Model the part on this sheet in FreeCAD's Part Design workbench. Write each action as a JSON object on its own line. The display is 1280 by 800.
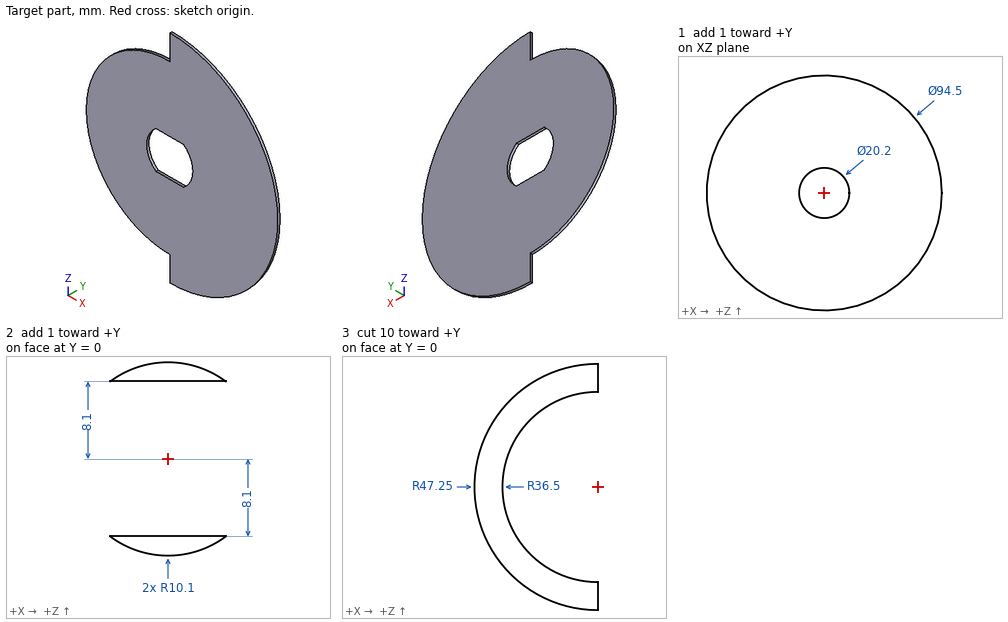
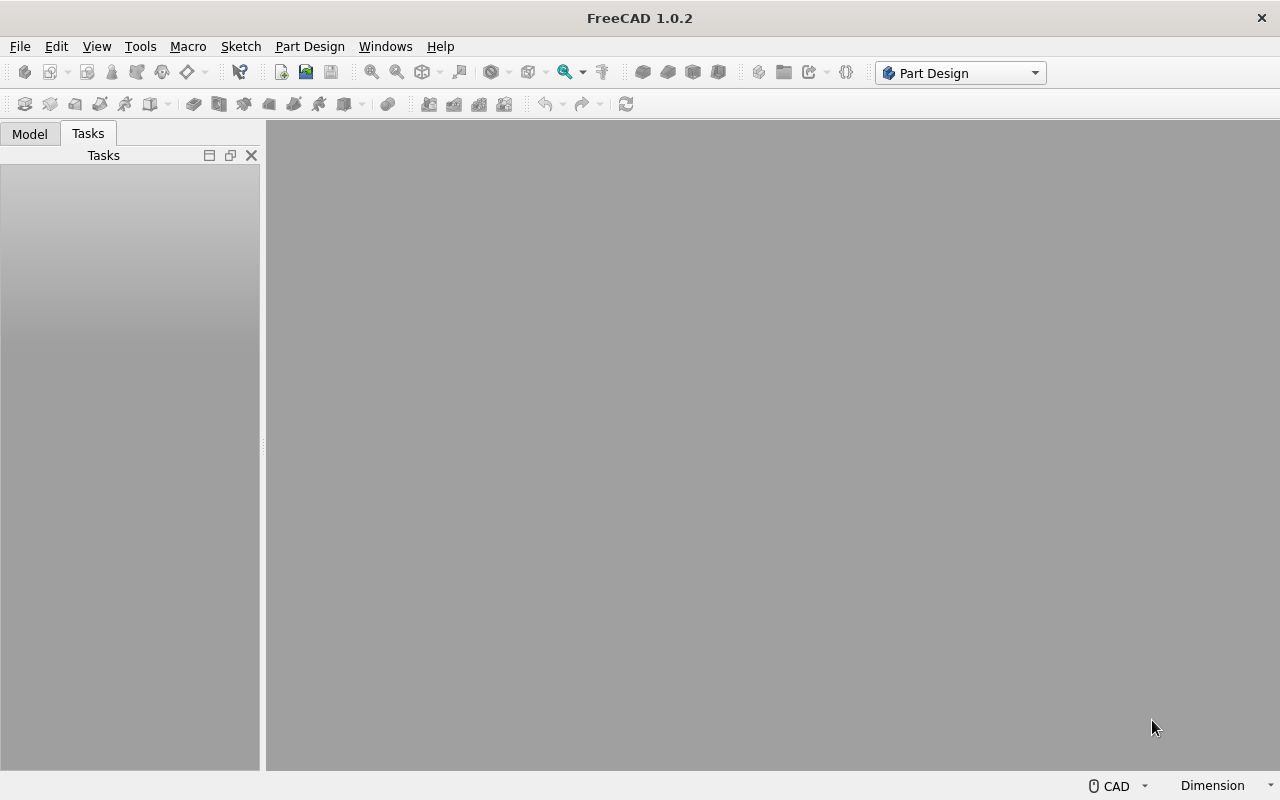
{"action": "left_click", "coordinate": [281, 72]}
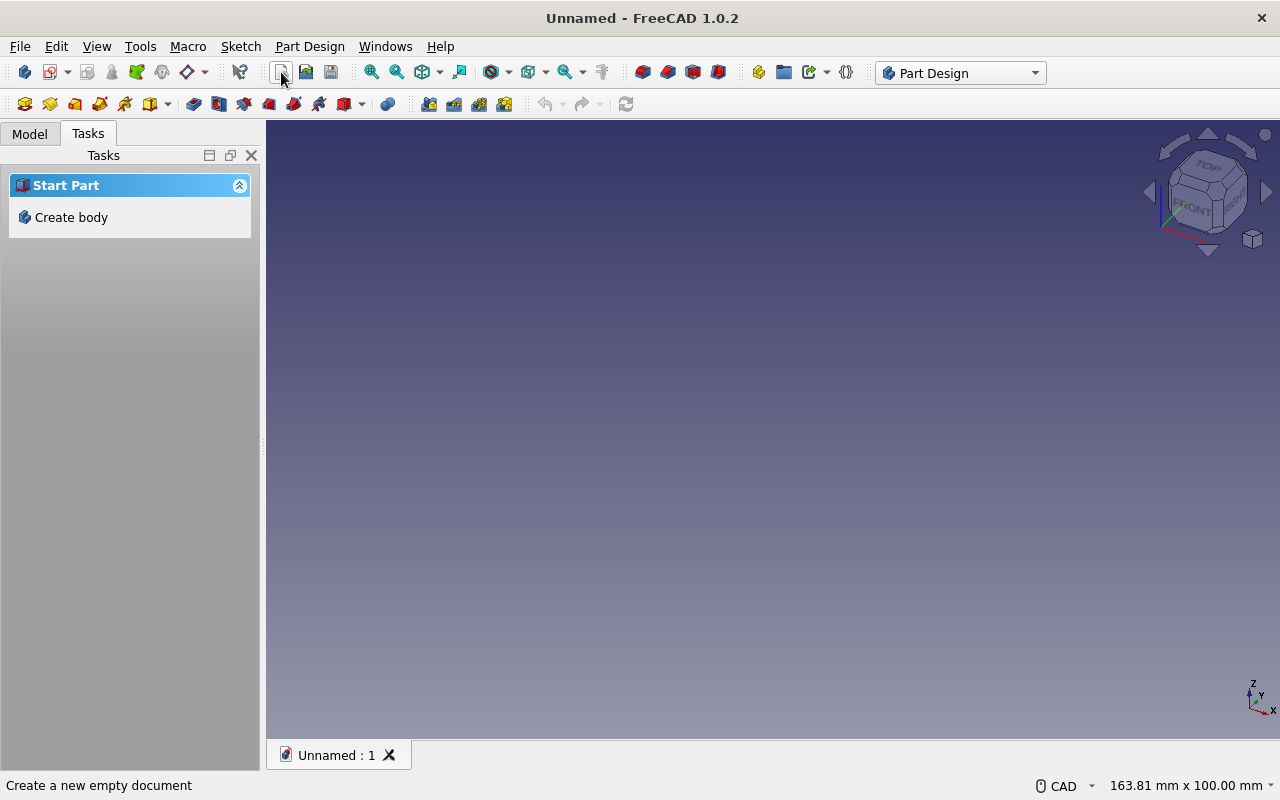
{"action": "left_click", "coordinate": [50, 72]}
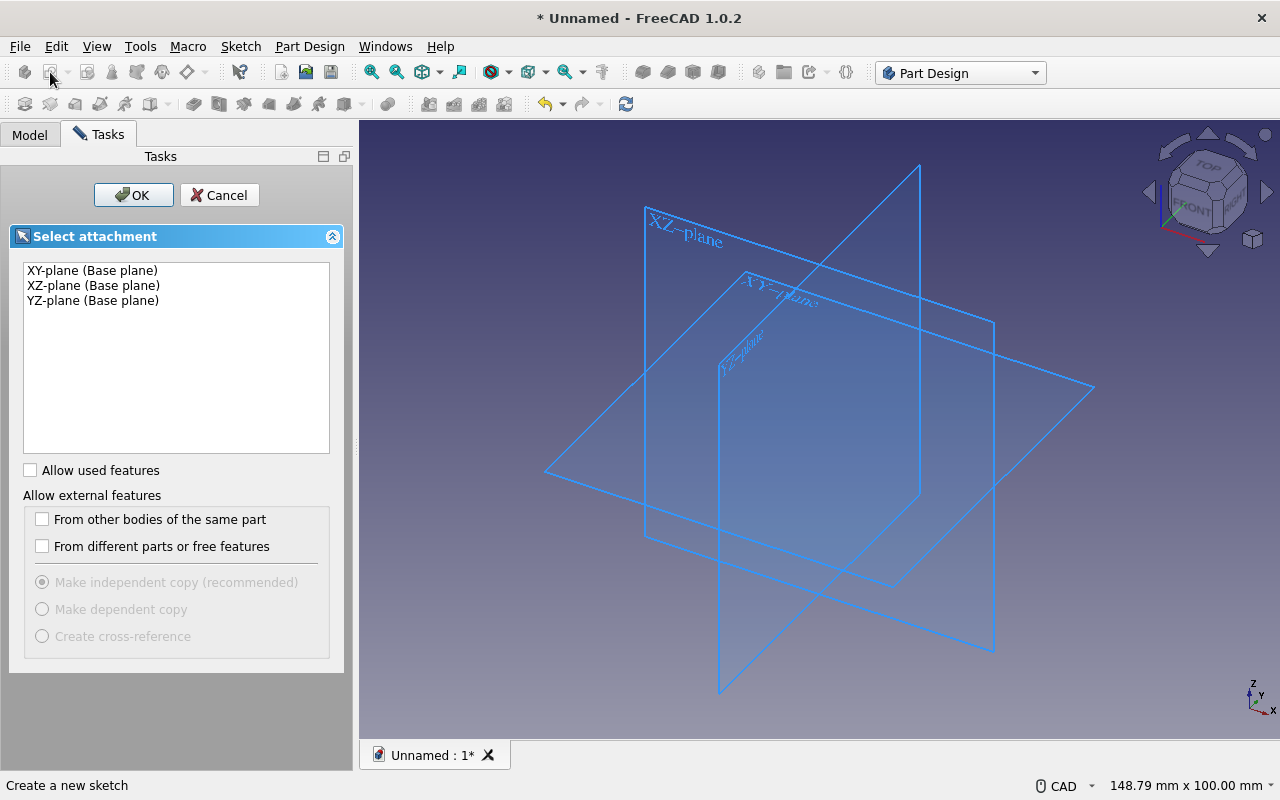
{"action": "left_click", "coordinate": [84, 286]}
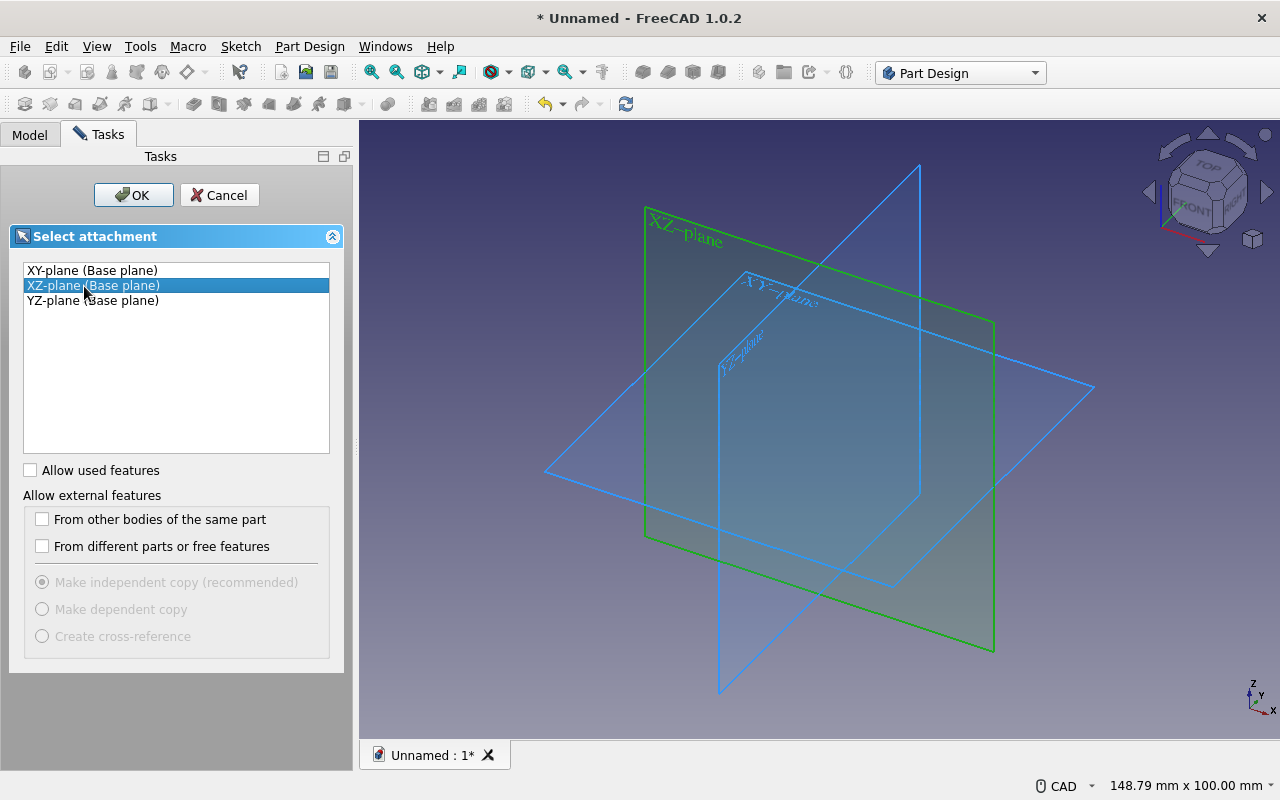
{"action": "left_click", "coordinate": [134, 195]}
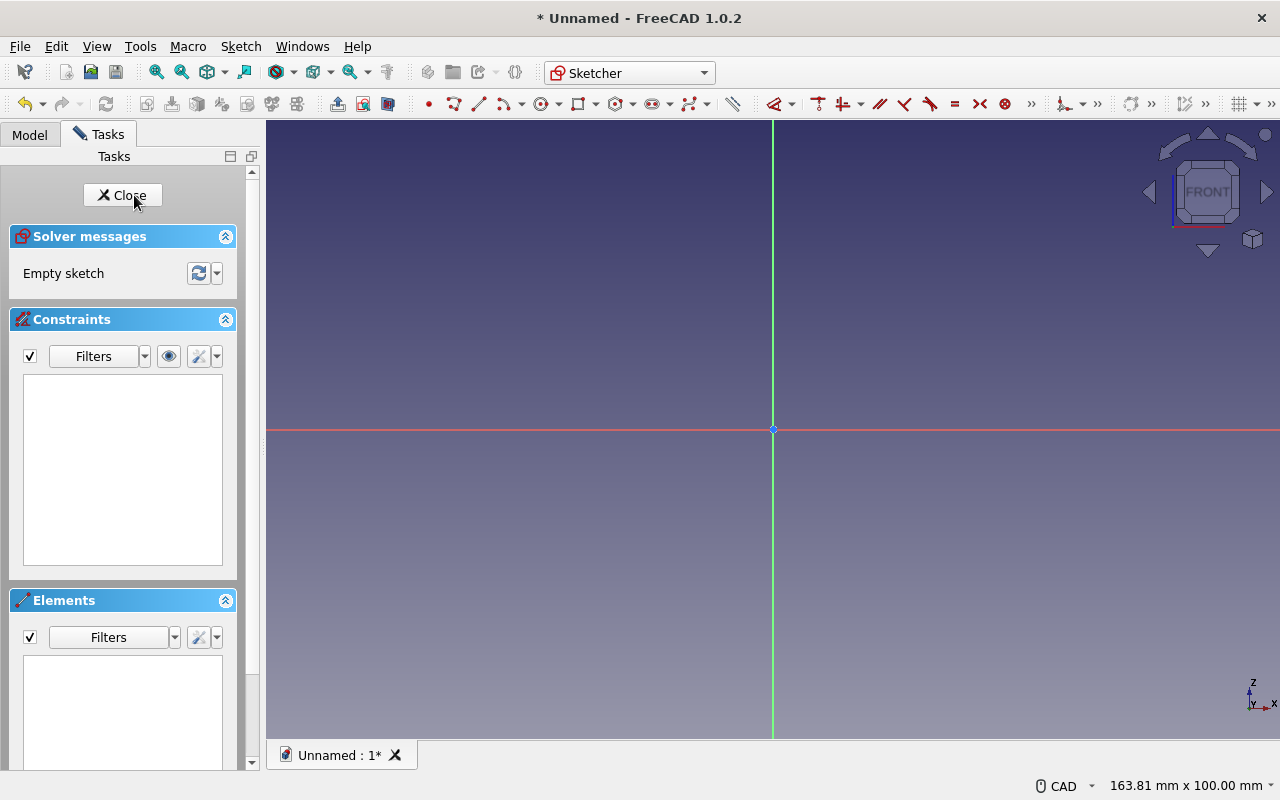
{"action": "scroll", "coordinate": [565, 429], "scroll_direction": "down", "scroll_amount": 2}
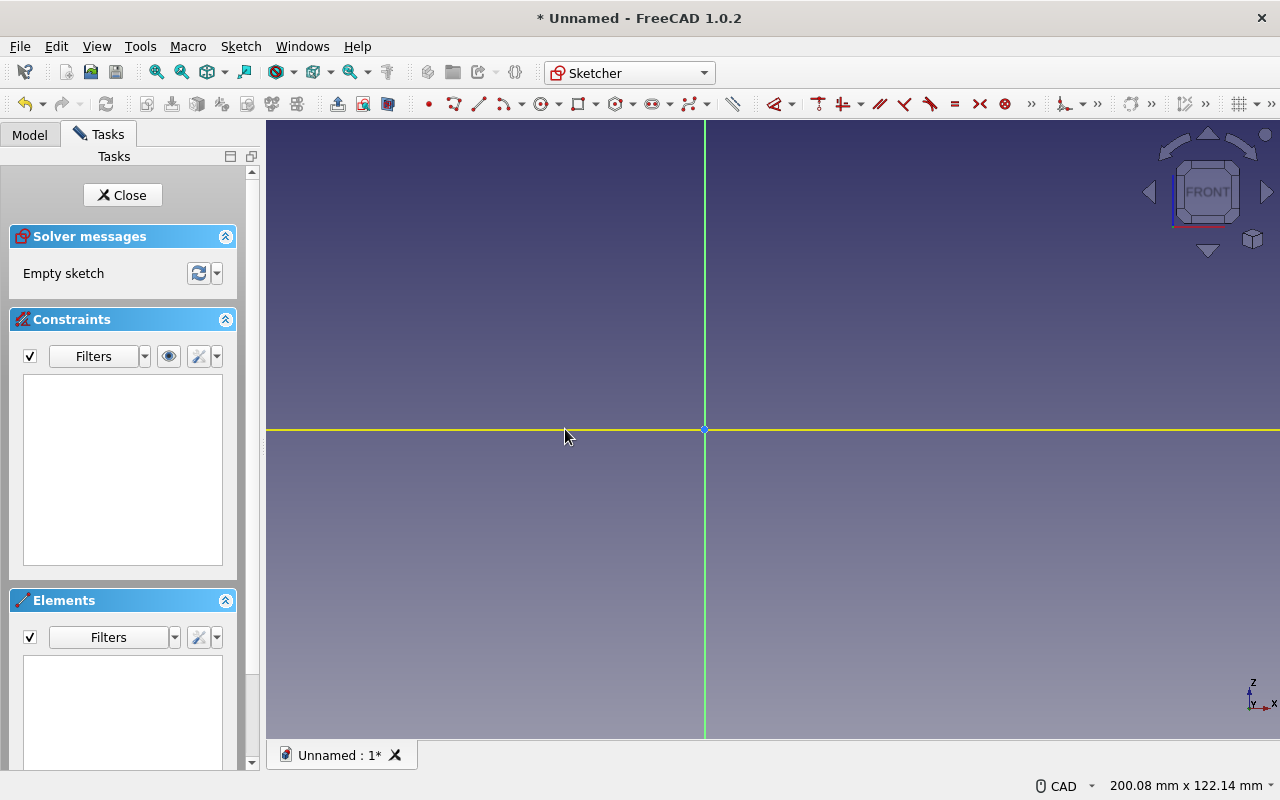
{"action": "left_click", "coordinate": [540, 104]}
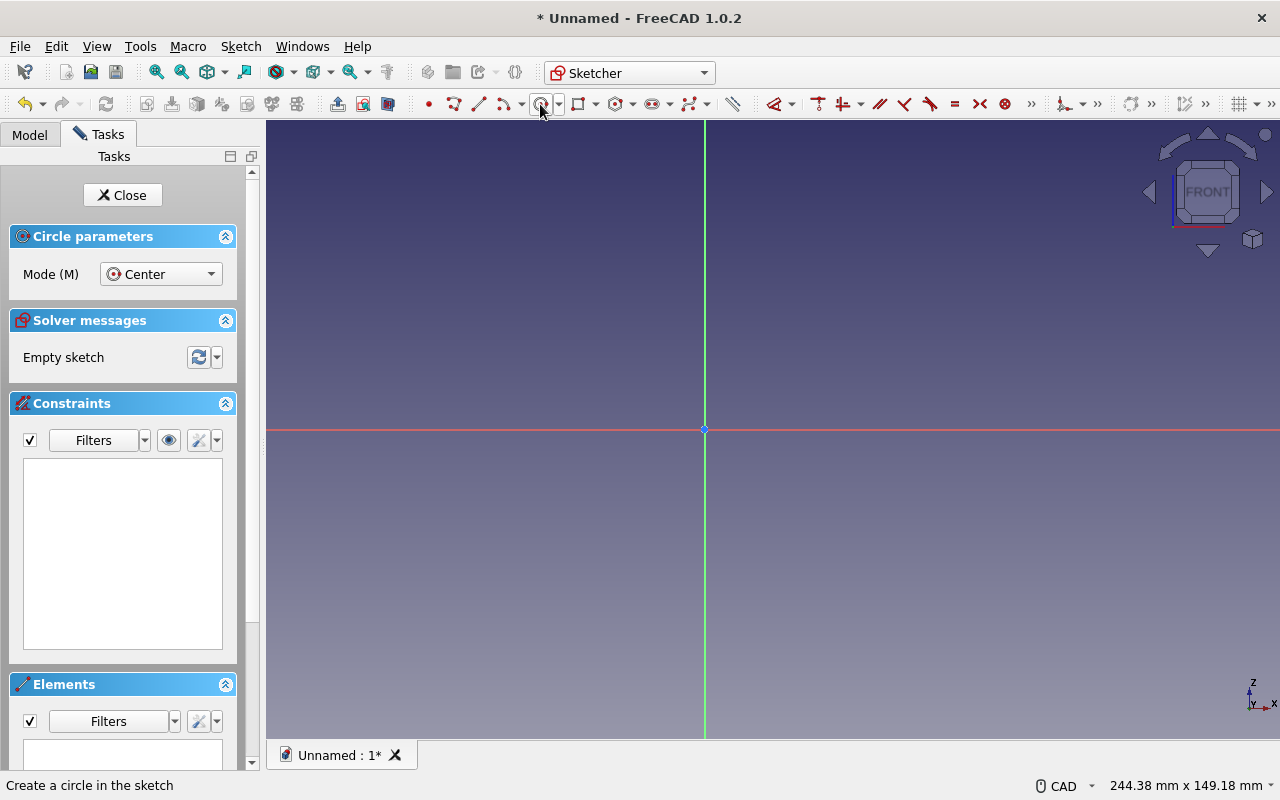
{"action": "left_click", "coordinate": [705, 430]}
{"action": "mouse_move", "coordinate": [843, 291]}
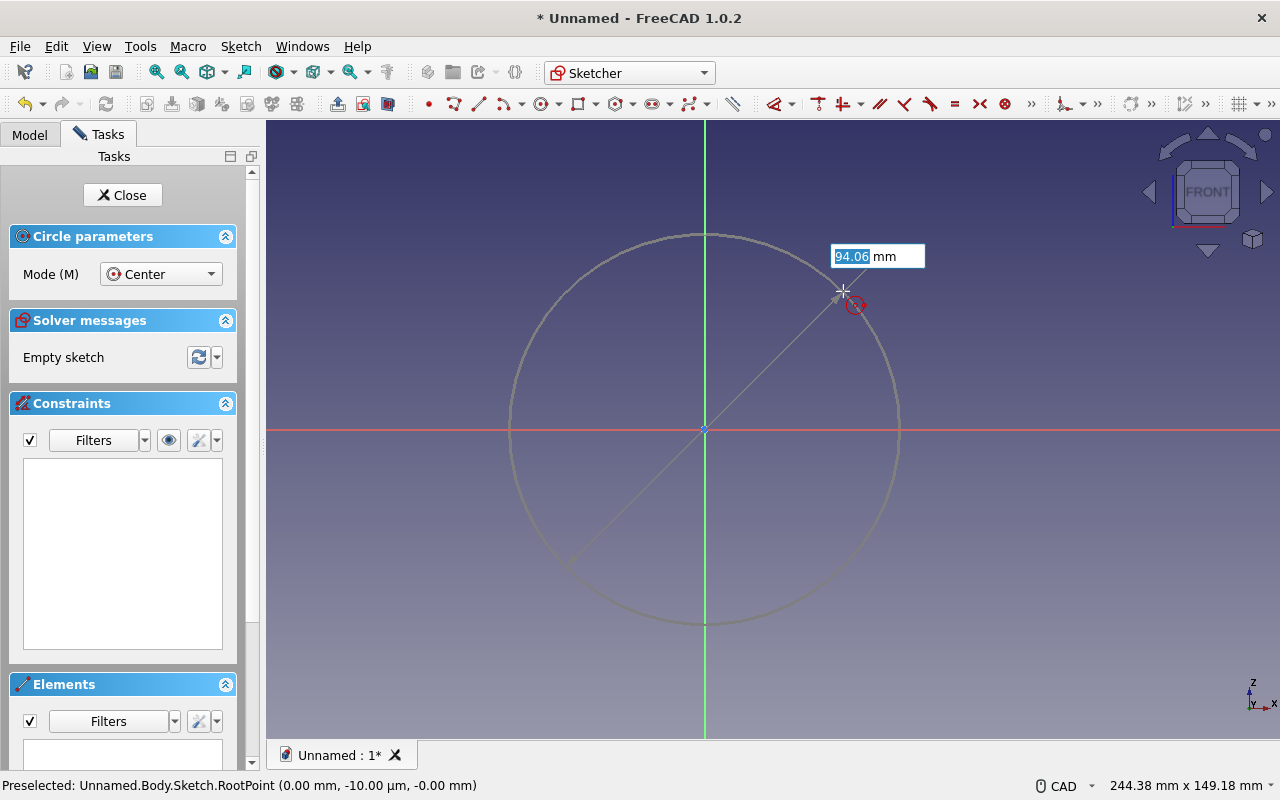
{"action": "type", "text": "94.5"}
{"action": "key", "text": "Return"}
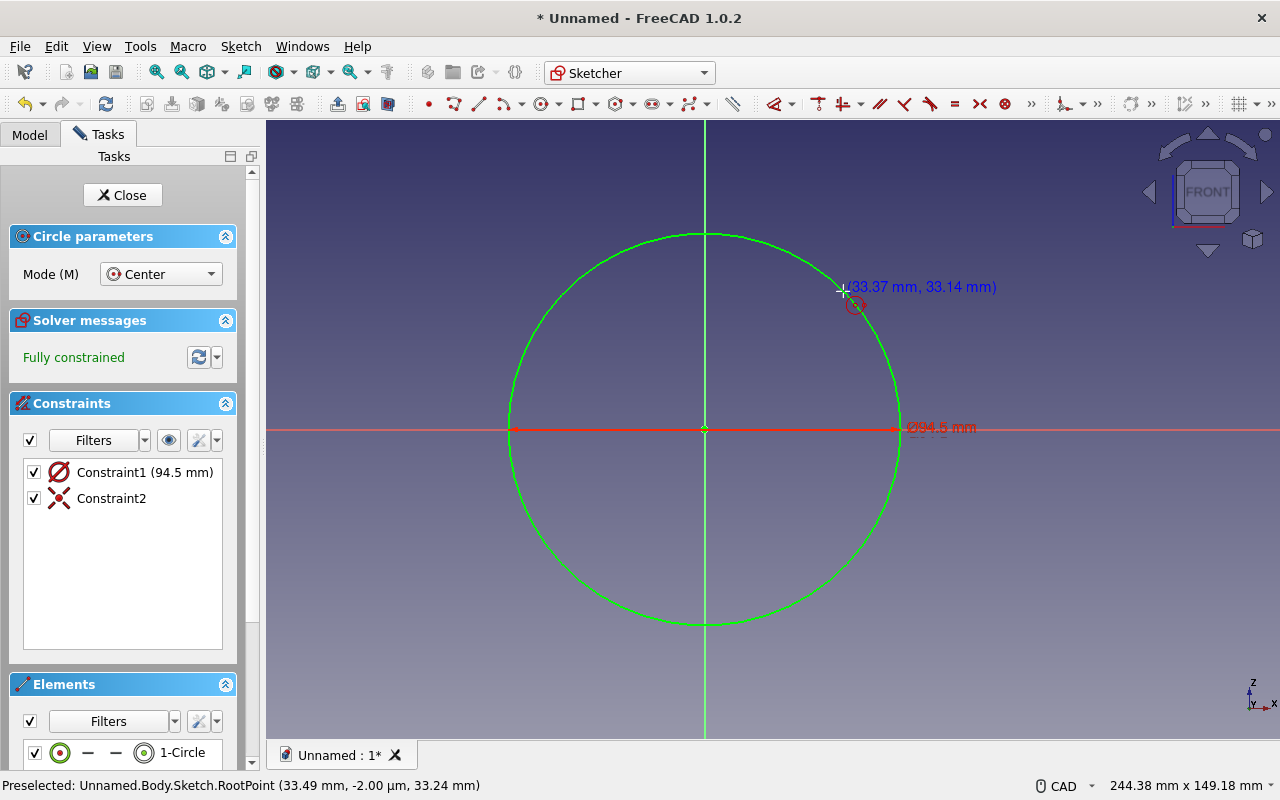
{"action": "left_click", "coordinate": [705, 430]}
{"action": "mouse_move", "coordinate": [734, 400]}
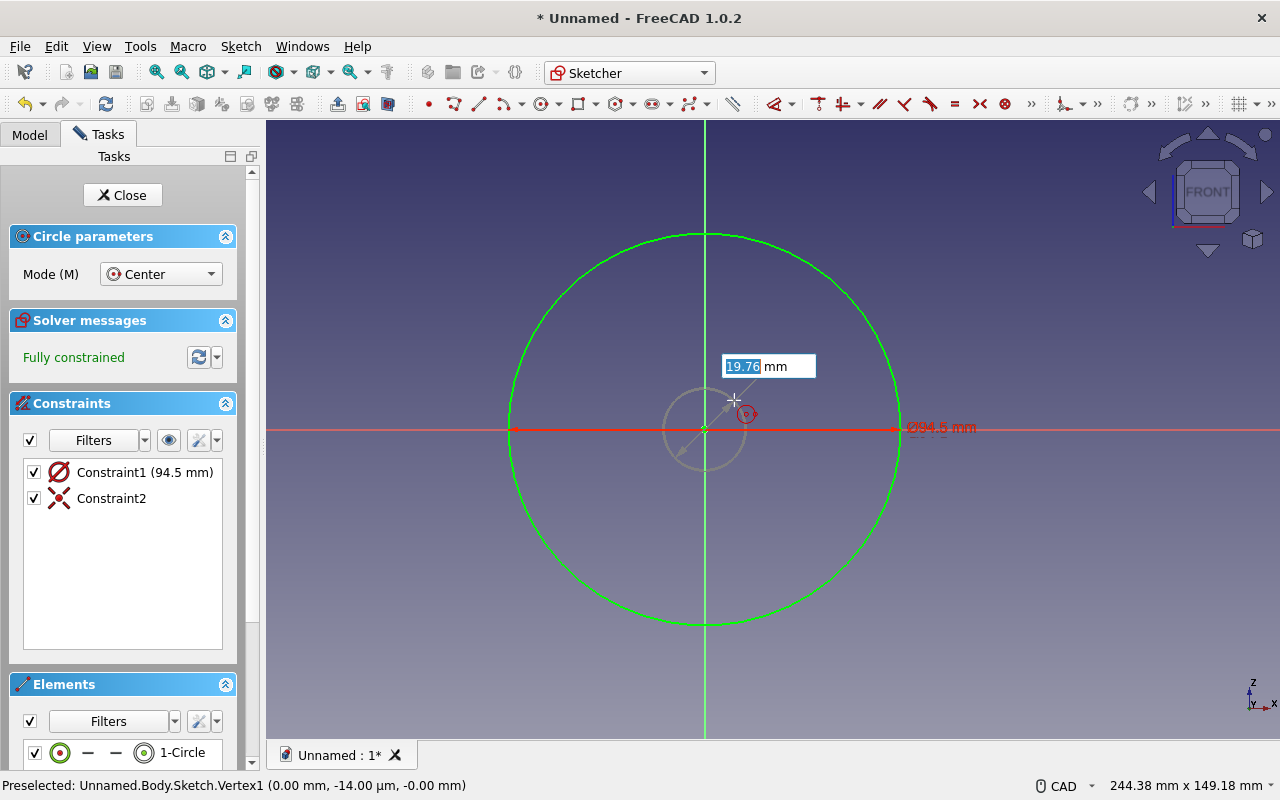
{"action": "type", "text": "20.2"}
{"action": "key", "text": "Return"}
{"action": "key", "text": "Escape"}